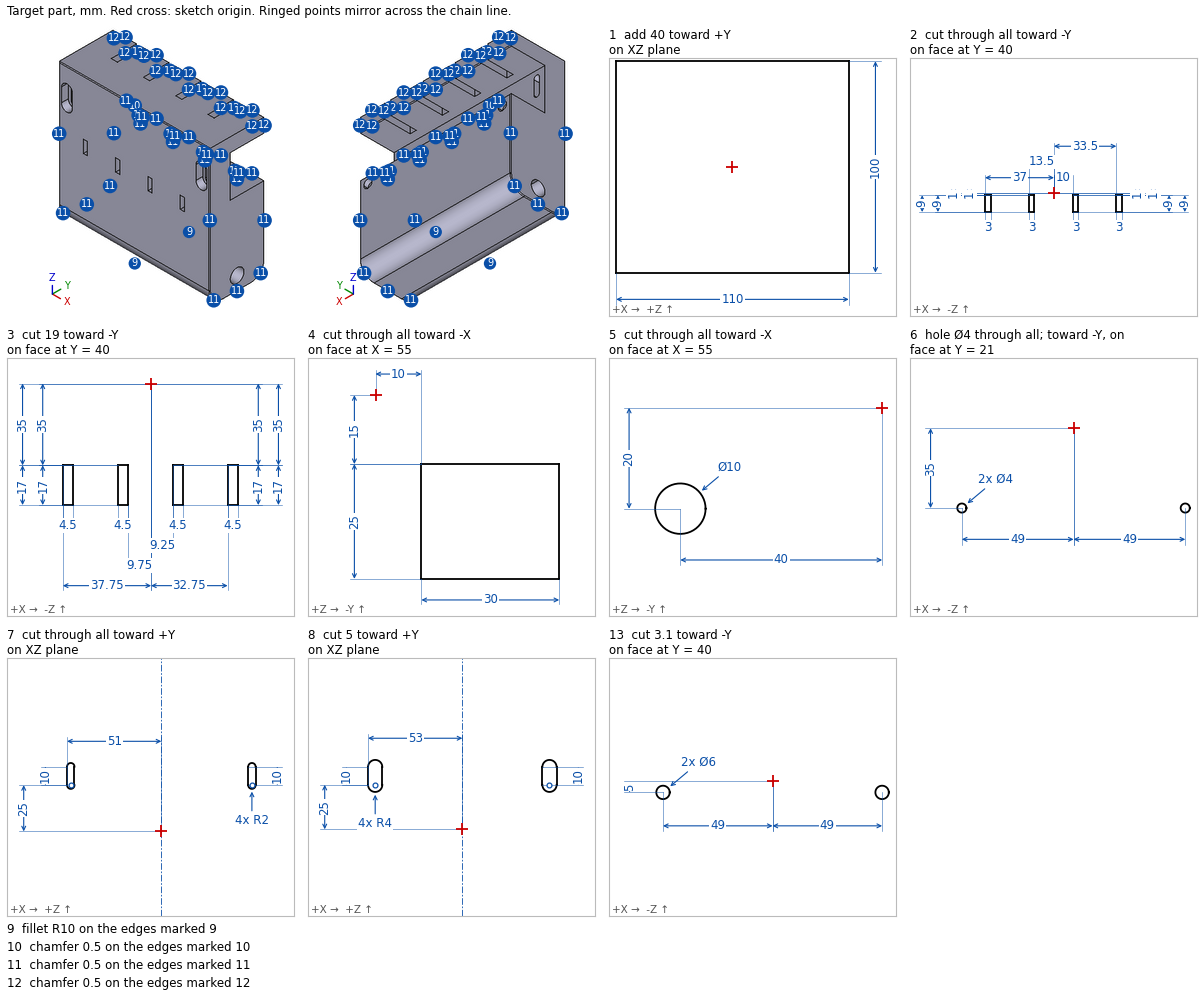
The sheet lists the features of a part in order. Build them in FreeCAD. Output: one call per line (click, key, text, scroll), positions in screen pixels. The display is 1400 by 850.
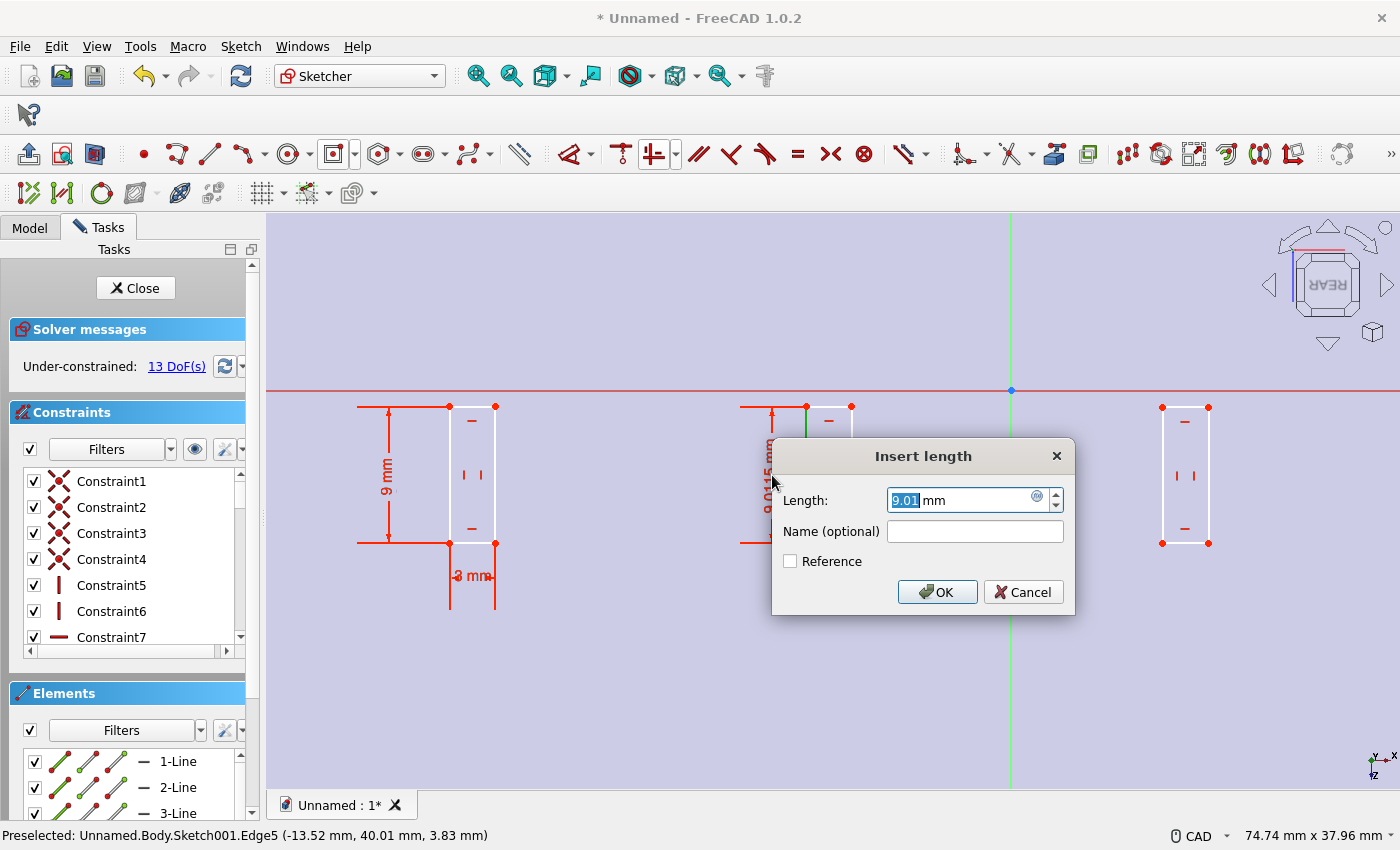
text(9)
key(Return)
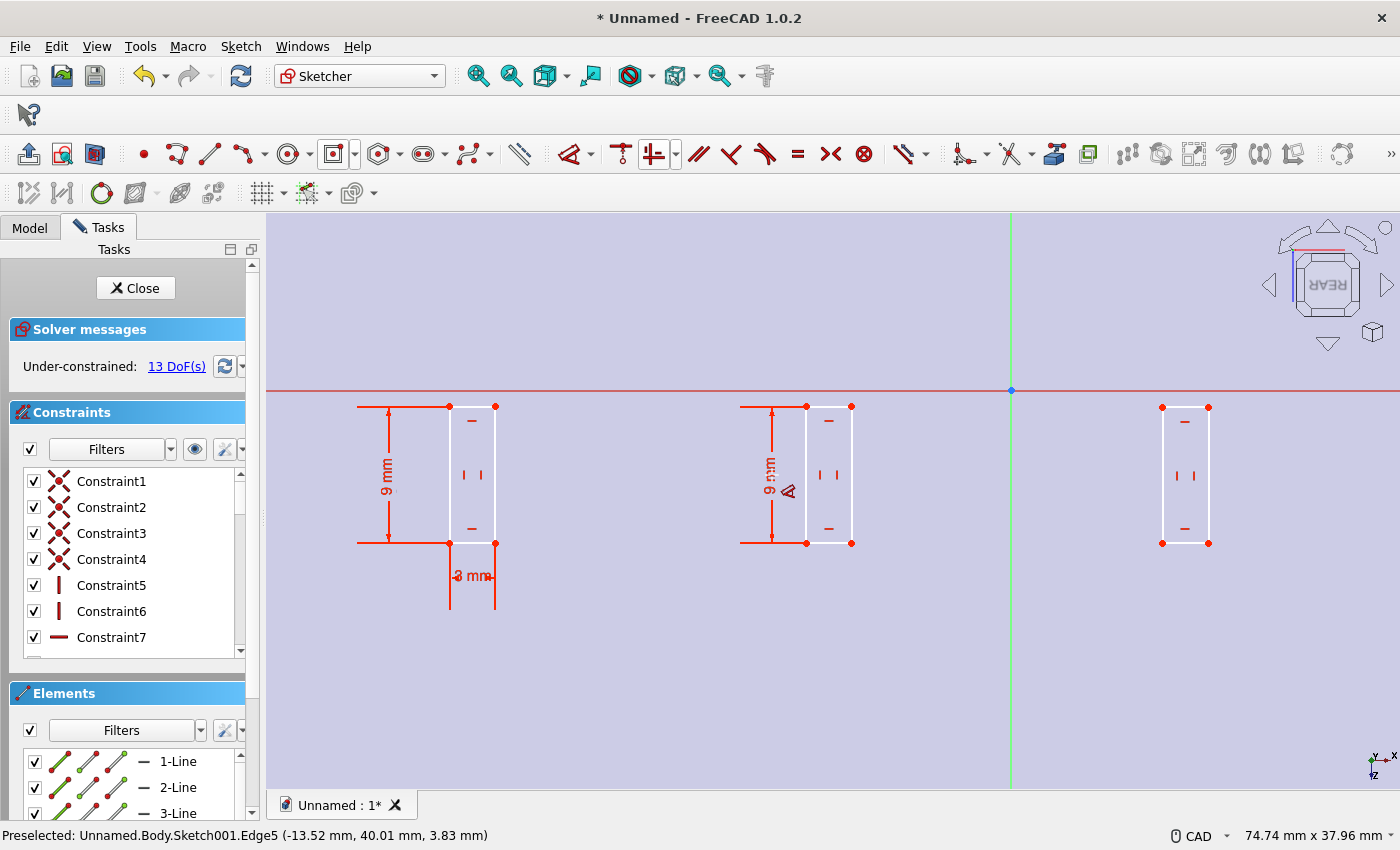
click(820, 543)
click(829, 577)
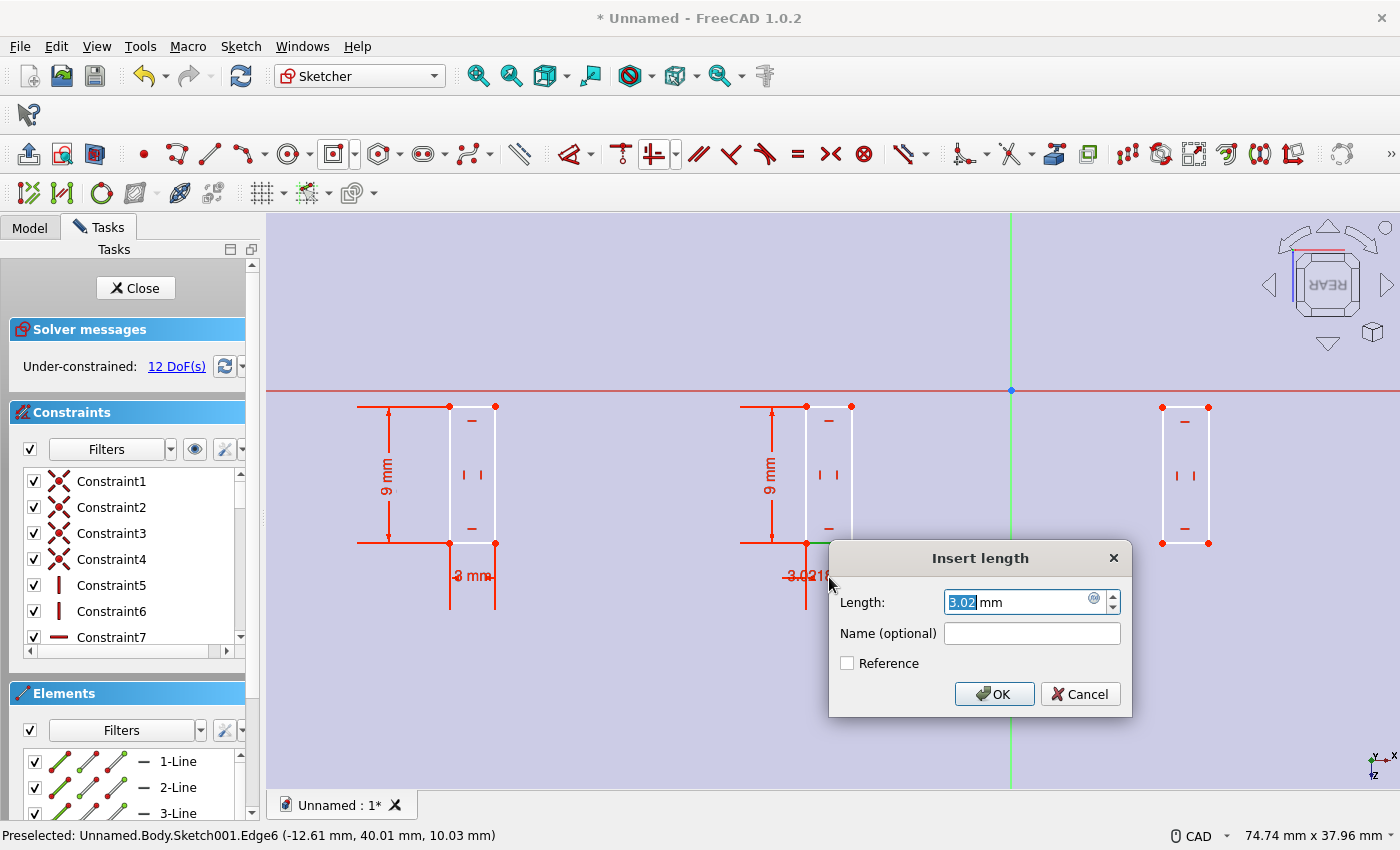
text(3)
key(Return)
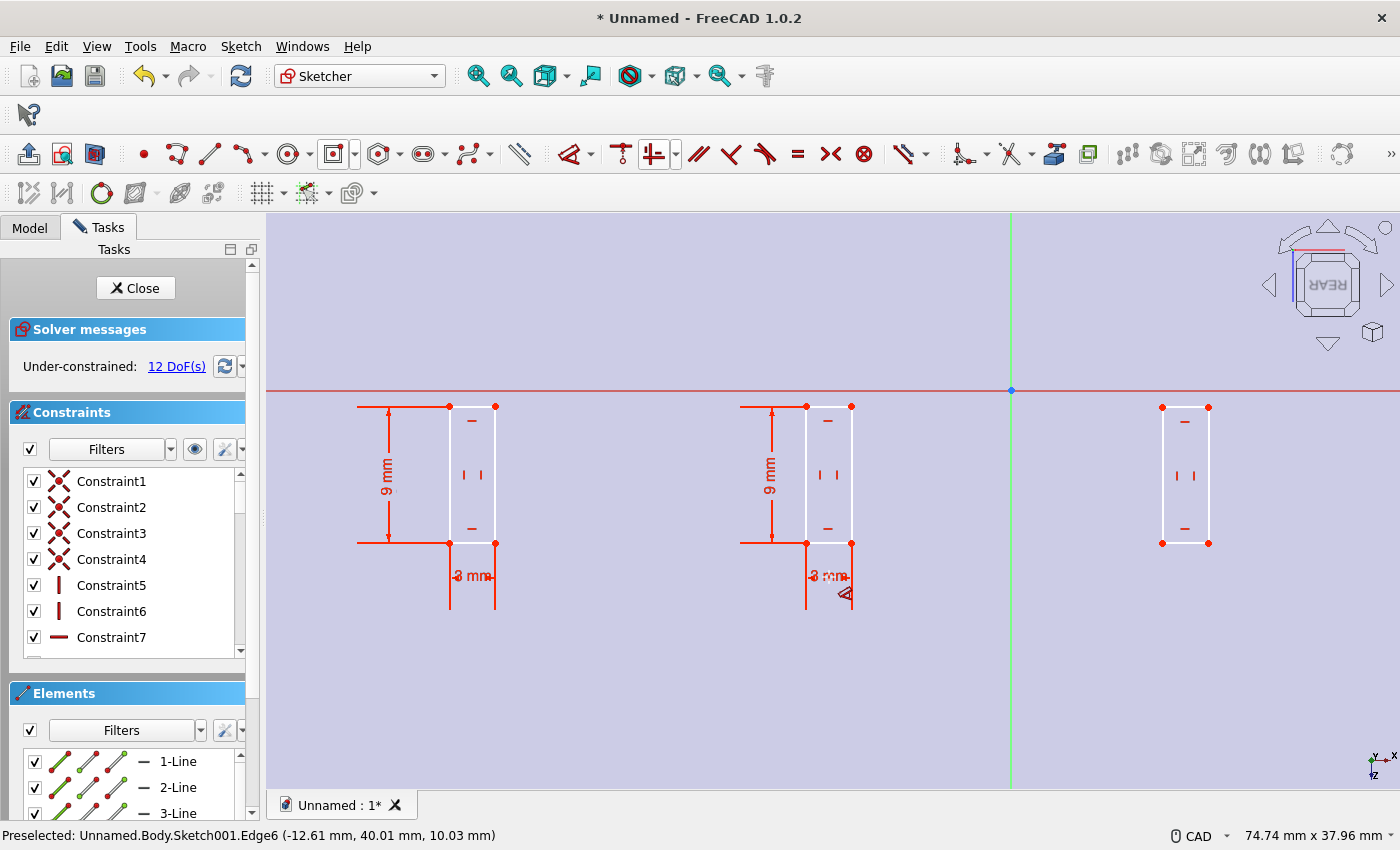
click(1163, 448)
click(1129, 475)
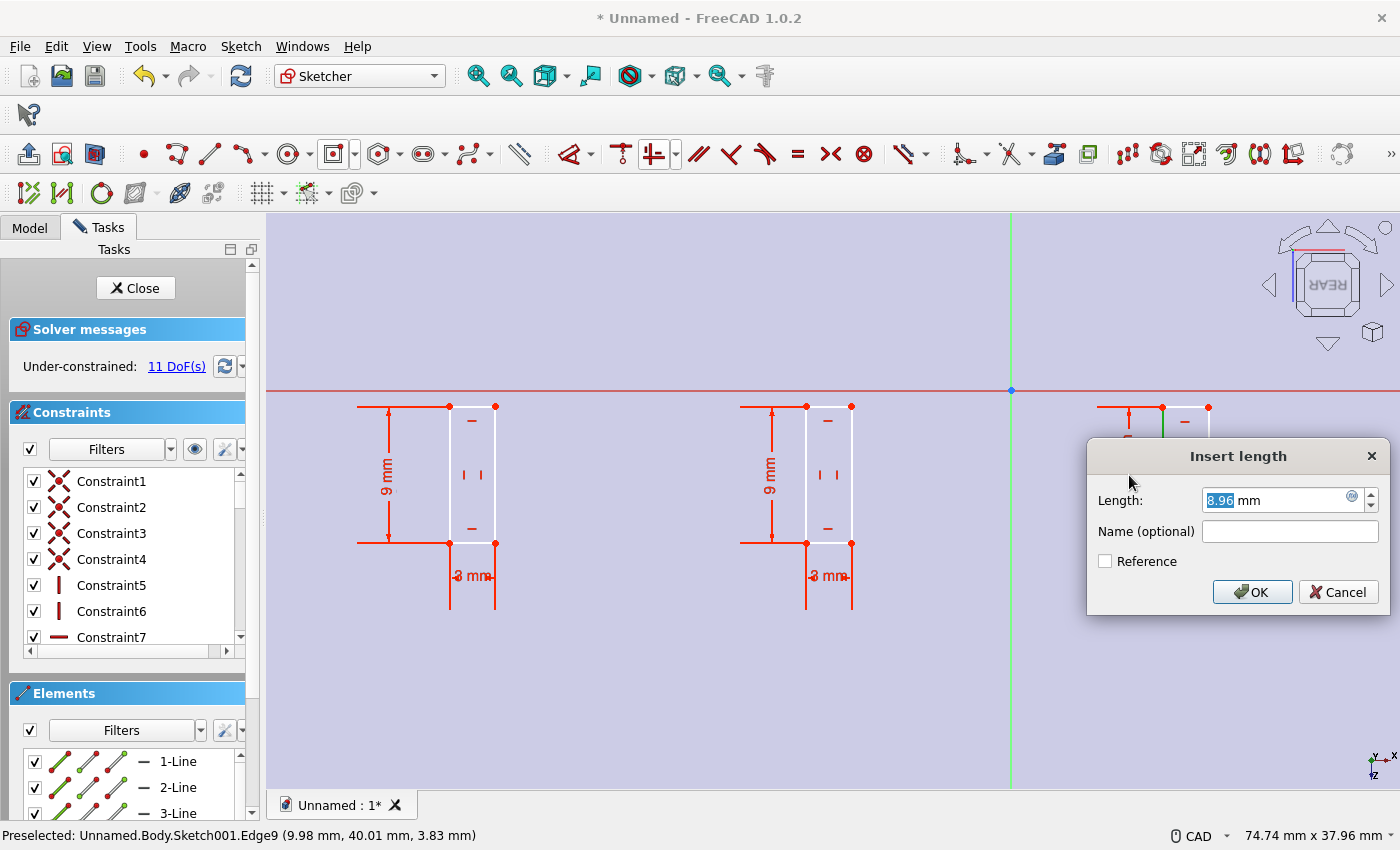
text(9)
key(Return)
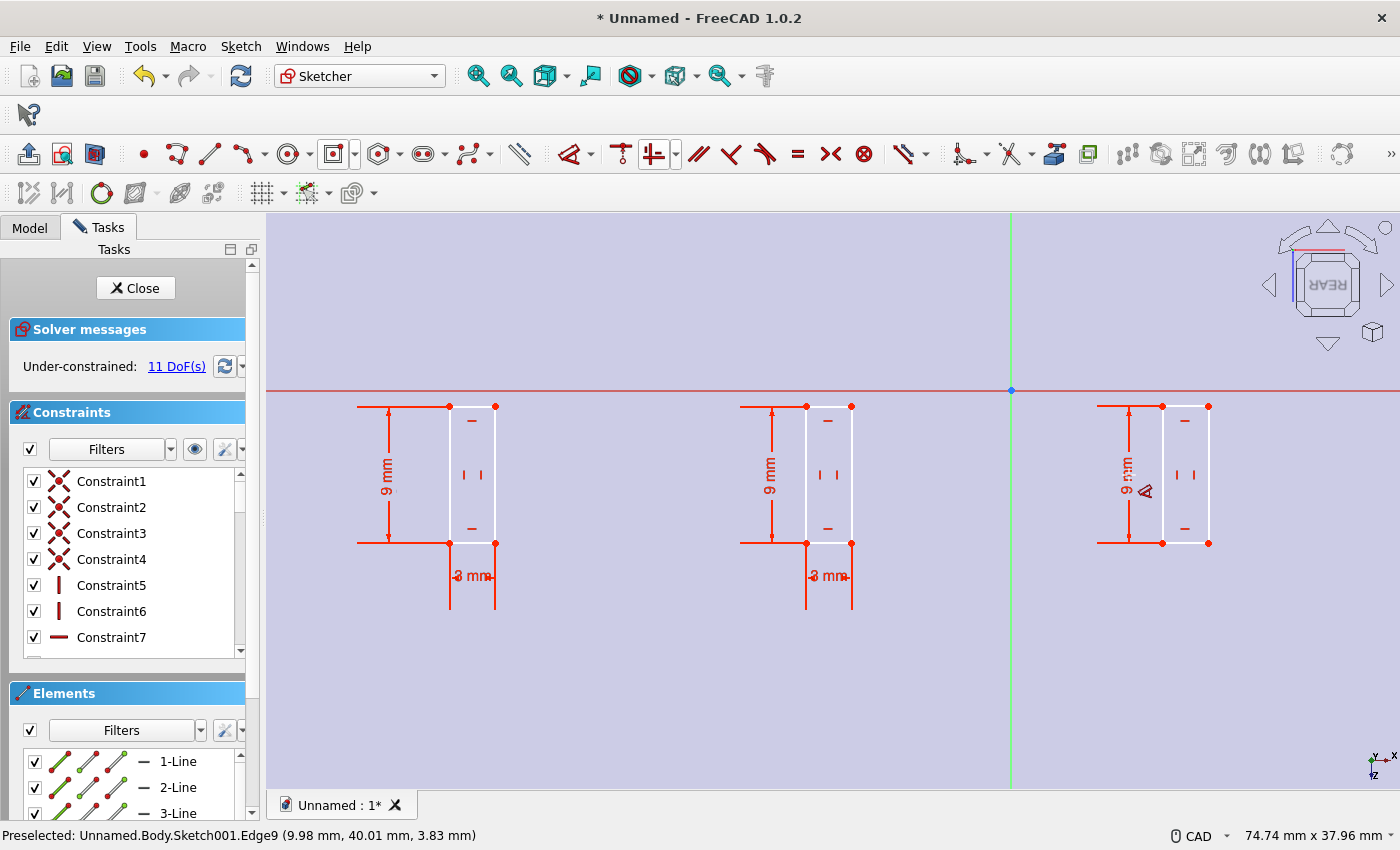
click(1177, 543)
click(1186, 577)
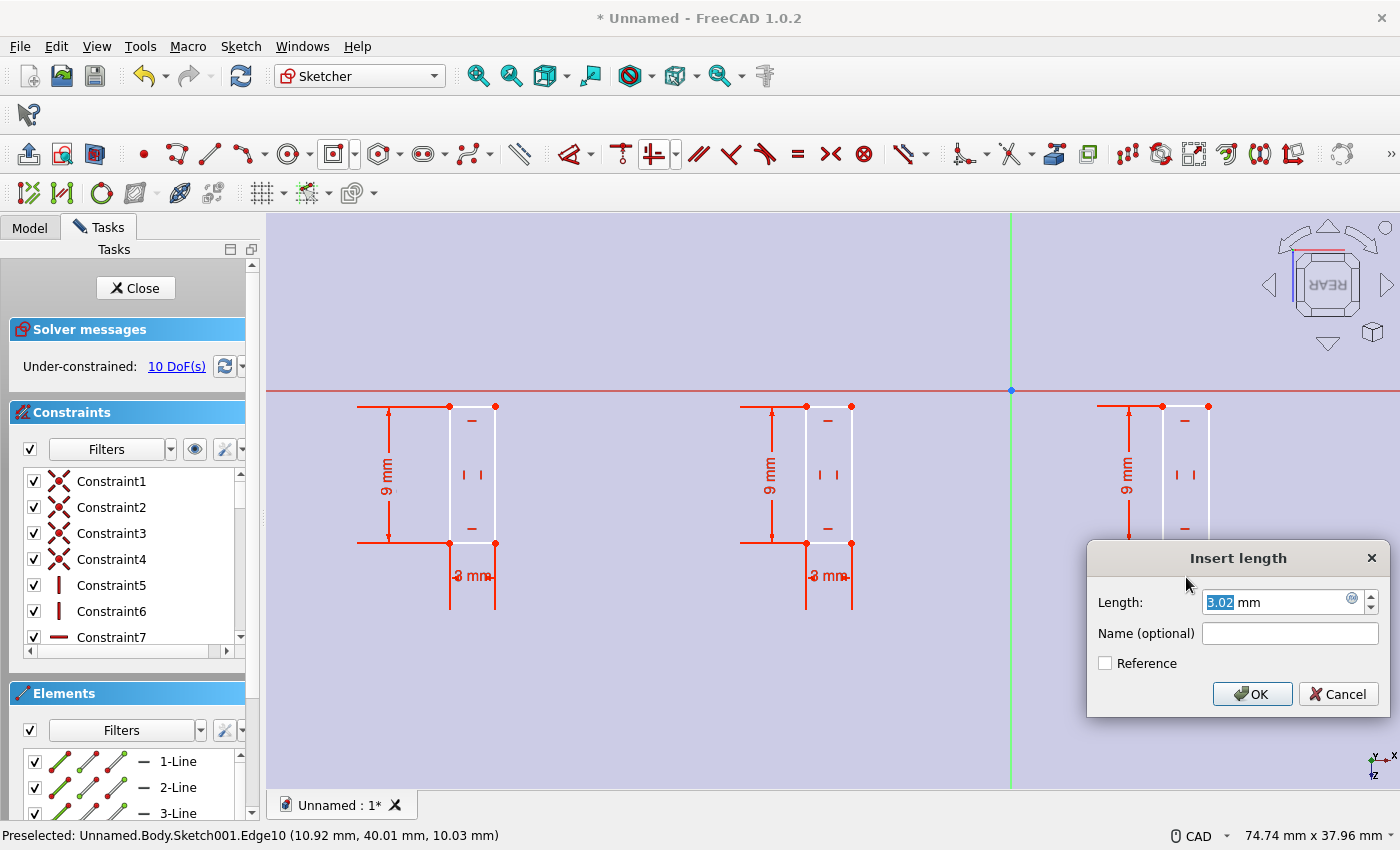
text(3)
key(Return)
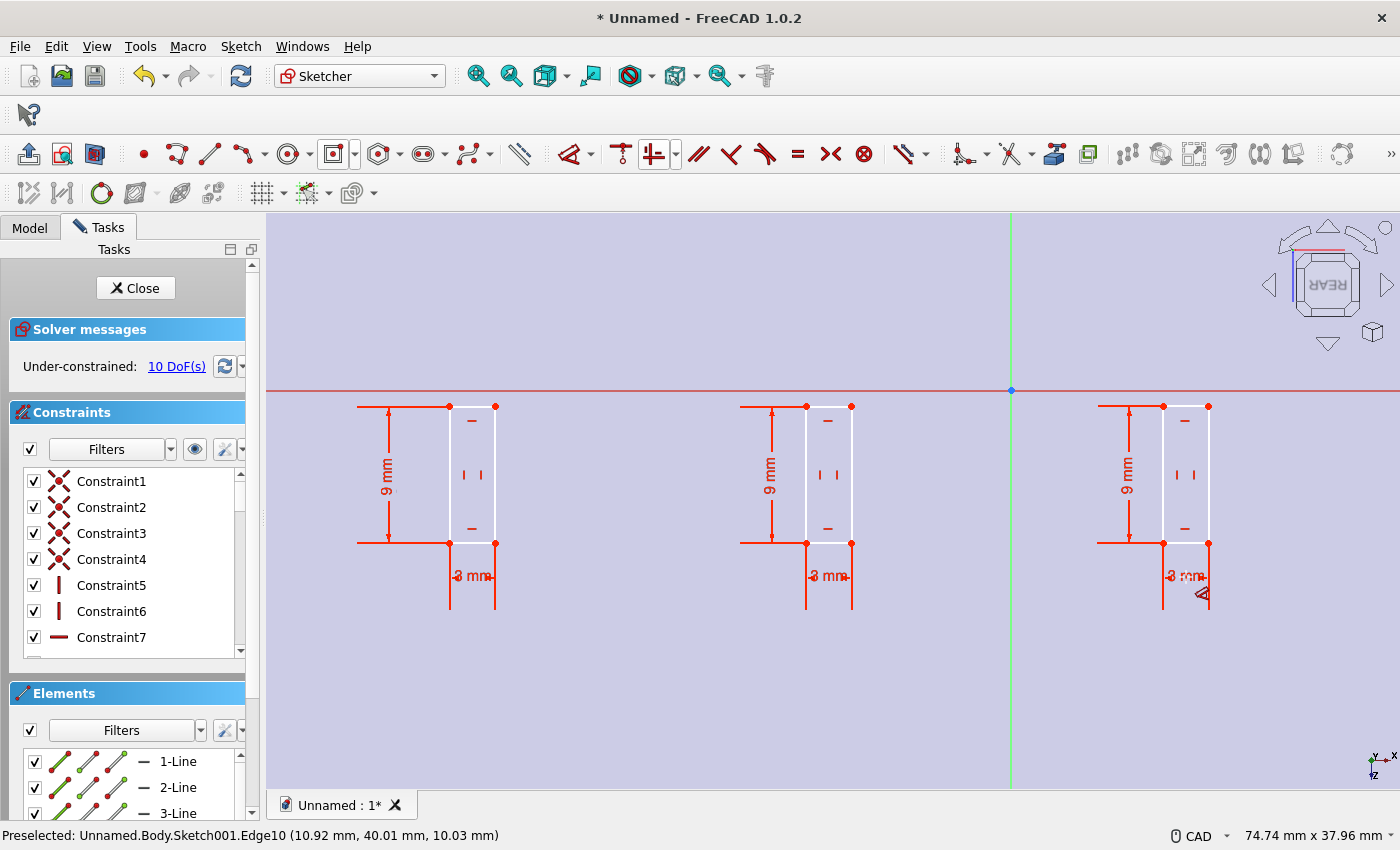
scroll(469, 543, down, 3)